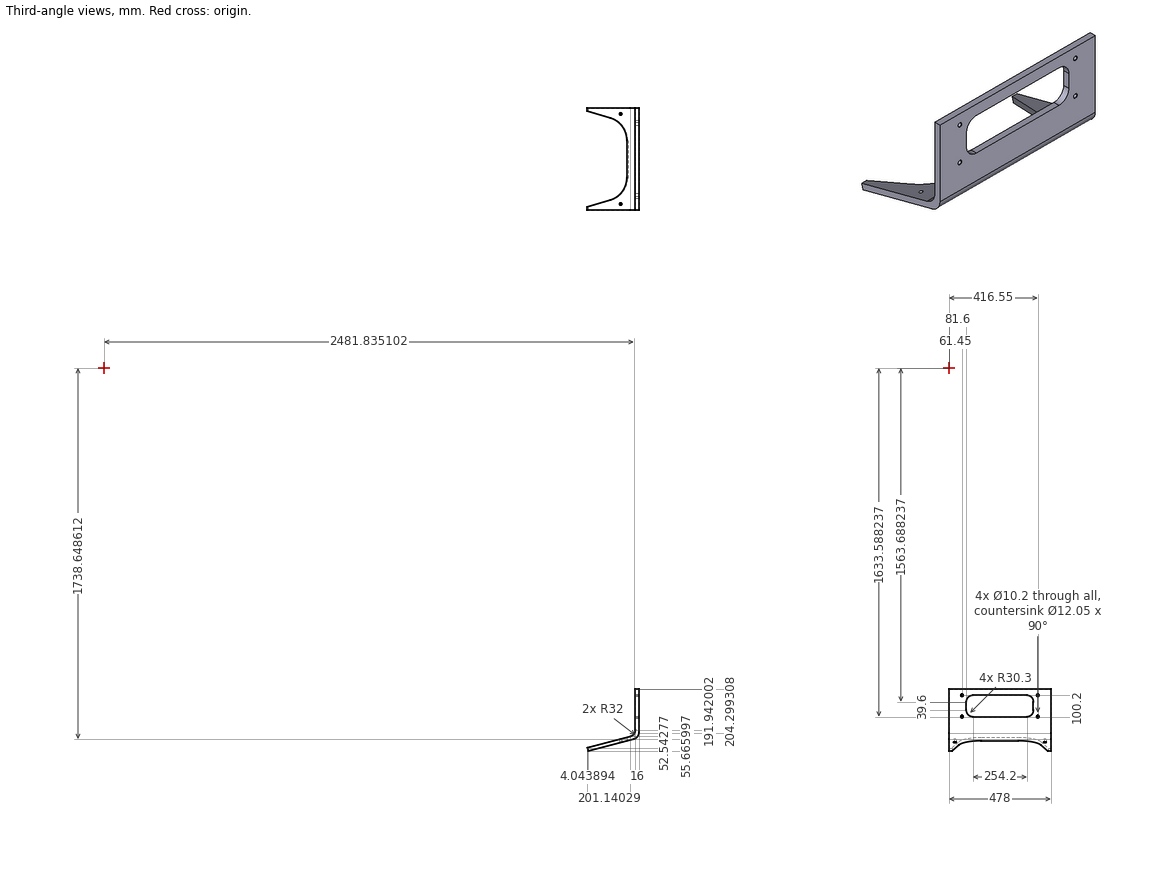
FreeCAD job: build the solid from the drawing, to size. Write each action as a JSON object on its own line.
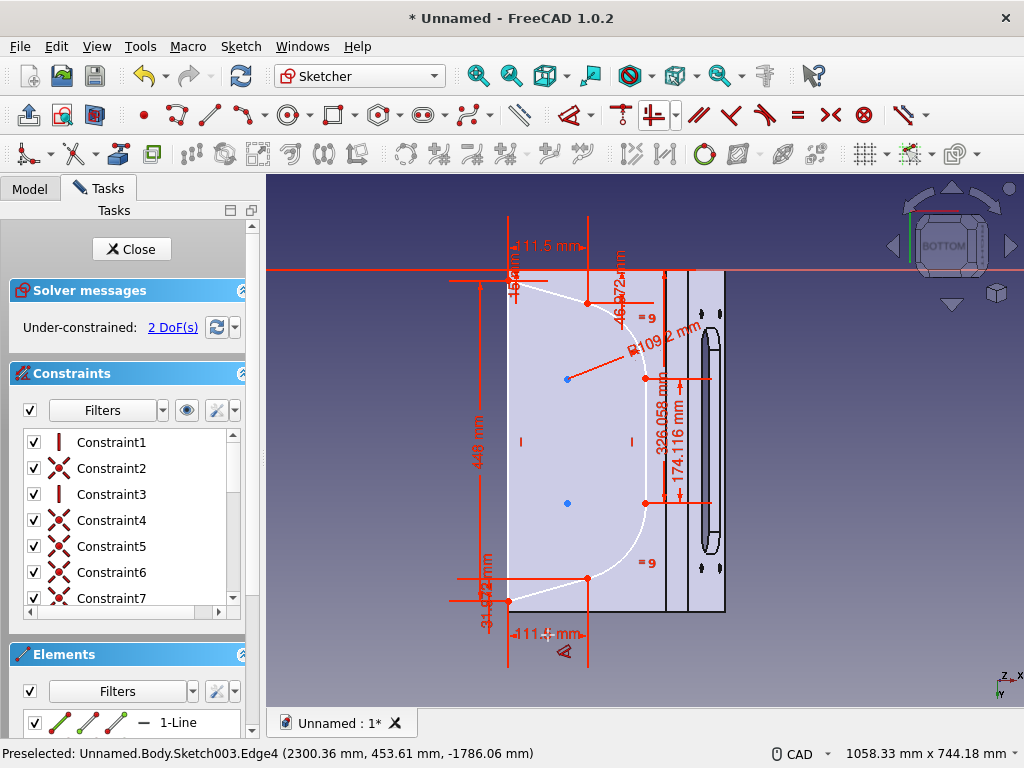
{"action": "left_click", "coordinate": [568, 379]}
{"action": "left_click", "coordinate": [602, 363]}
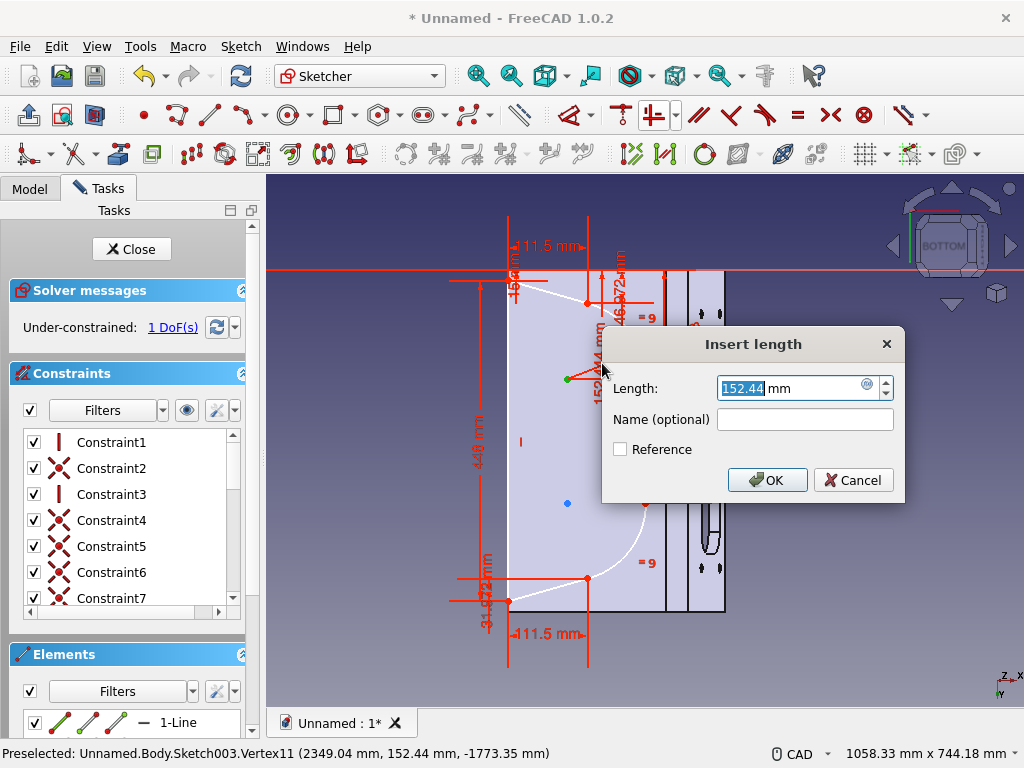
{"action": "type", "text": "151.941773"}
{"action": "key", "text": "Return"}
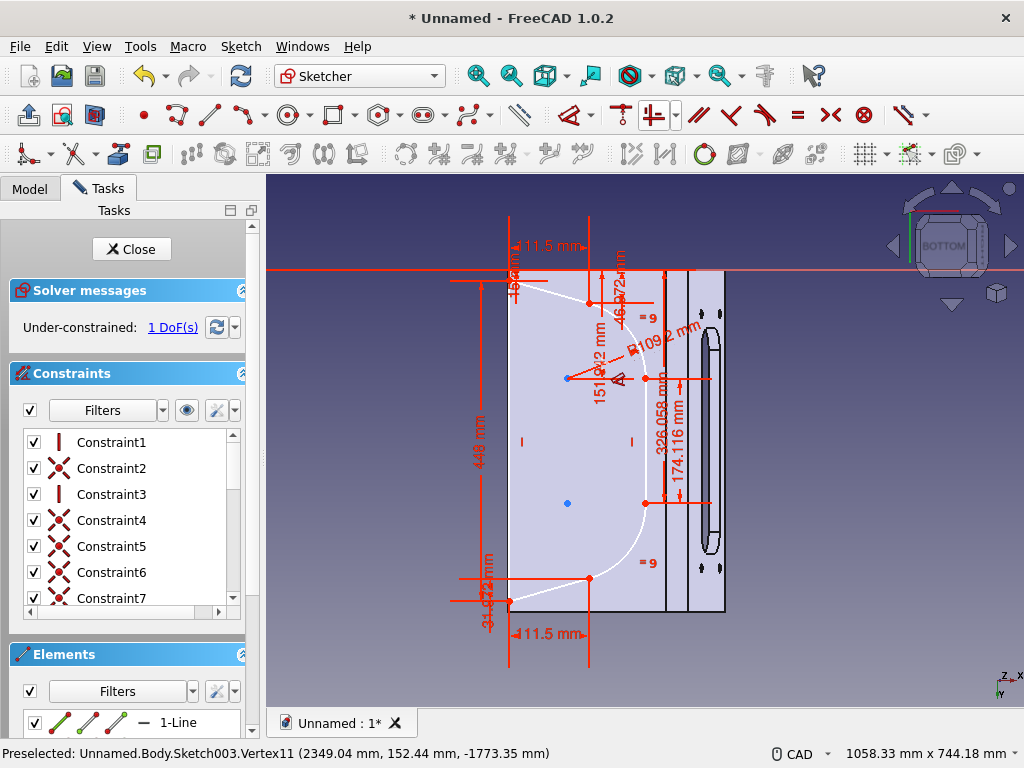
{"action": "left_click", "coordinate": [646, 503]}
{"action": "left_click", "coordinate": [470, 236]}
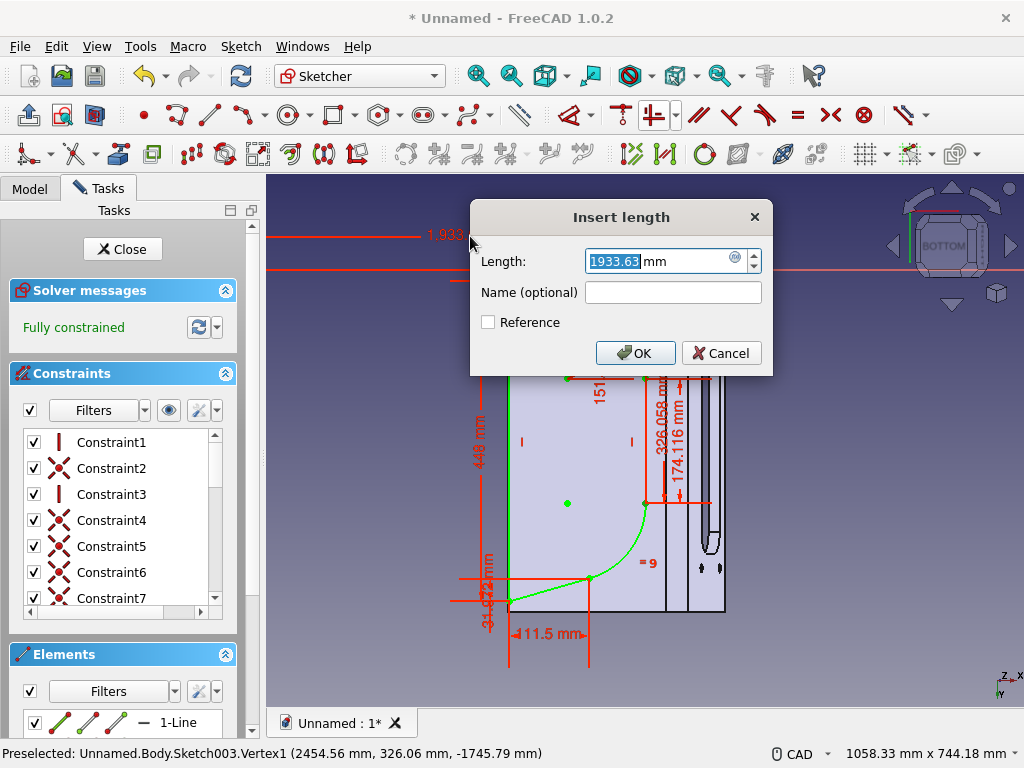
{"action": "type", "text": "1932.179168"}
{"action": "key", "text": "Return"}
{"action": "key", "text": "Escape"}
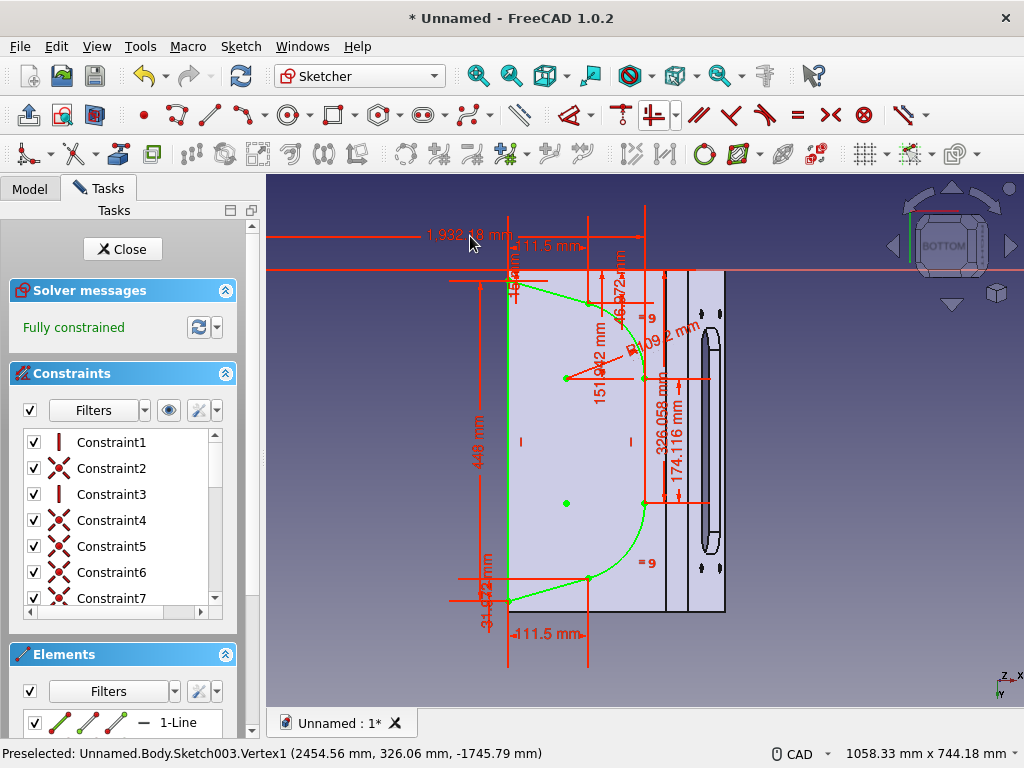
{"action": "left_click", "coordinate": [123, 249]}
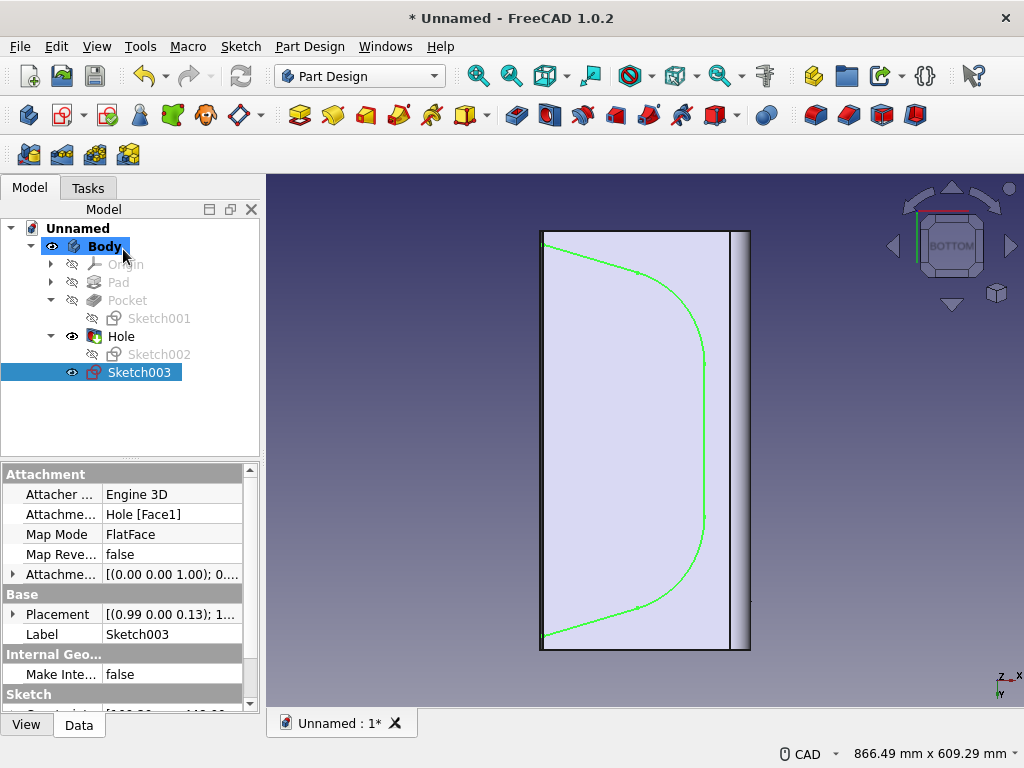
{"action": "left_click", "coordinate": [517, 116]}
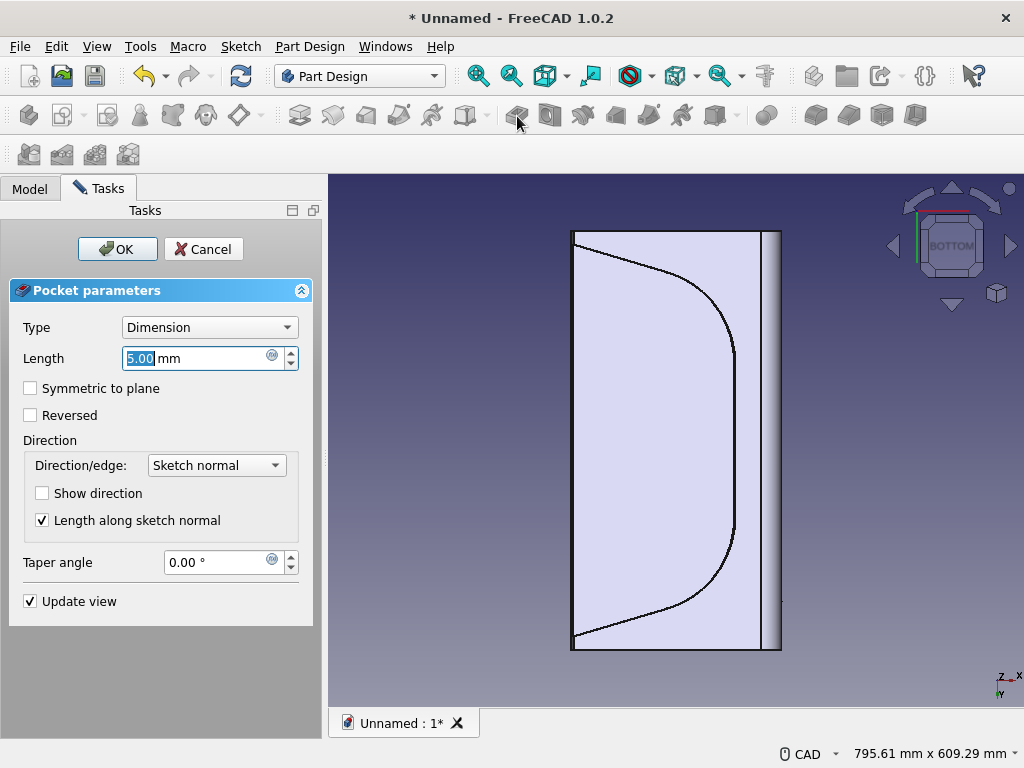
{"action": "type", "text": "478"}
{"action": "key", "text": "Tab"}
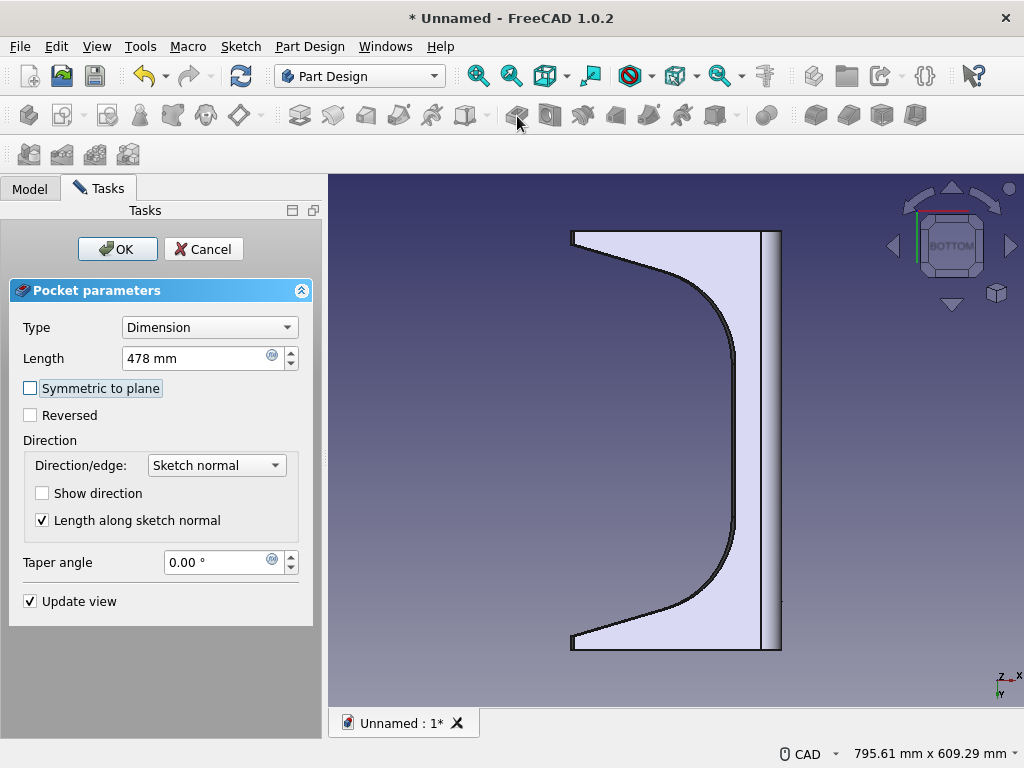
{"action": "left_click", "coordinate": [118, 249]}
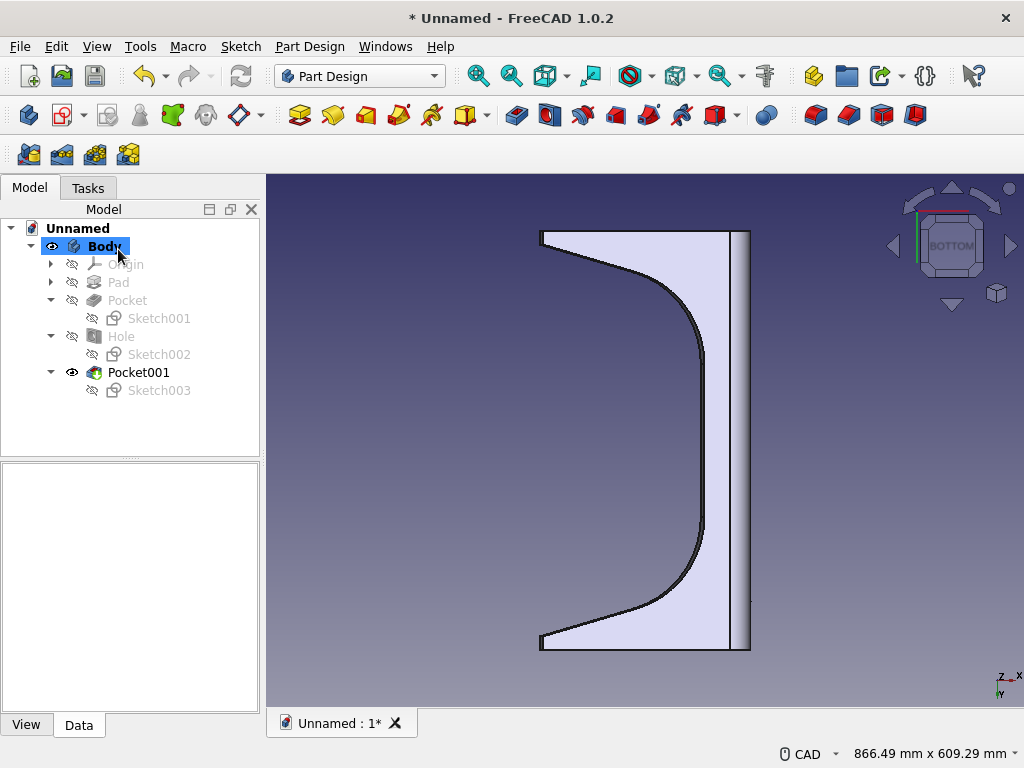
{"action": "left_click", "coordinate": [690, 260]}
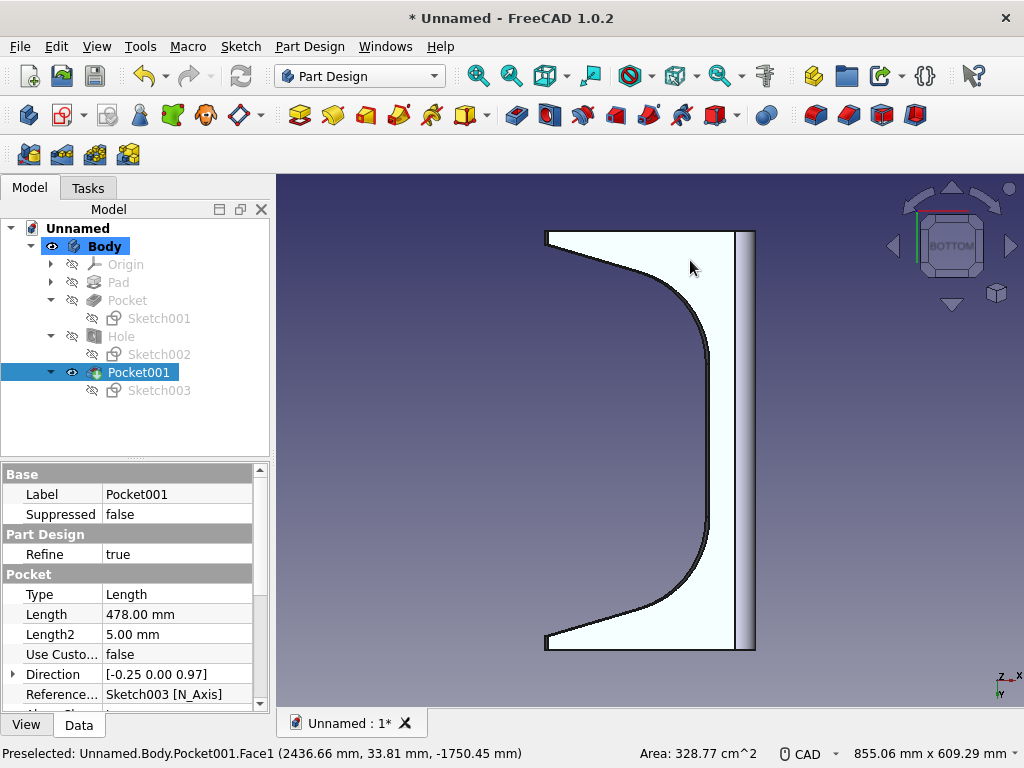
{"action": "left_click", "coordinate": [62, 116]}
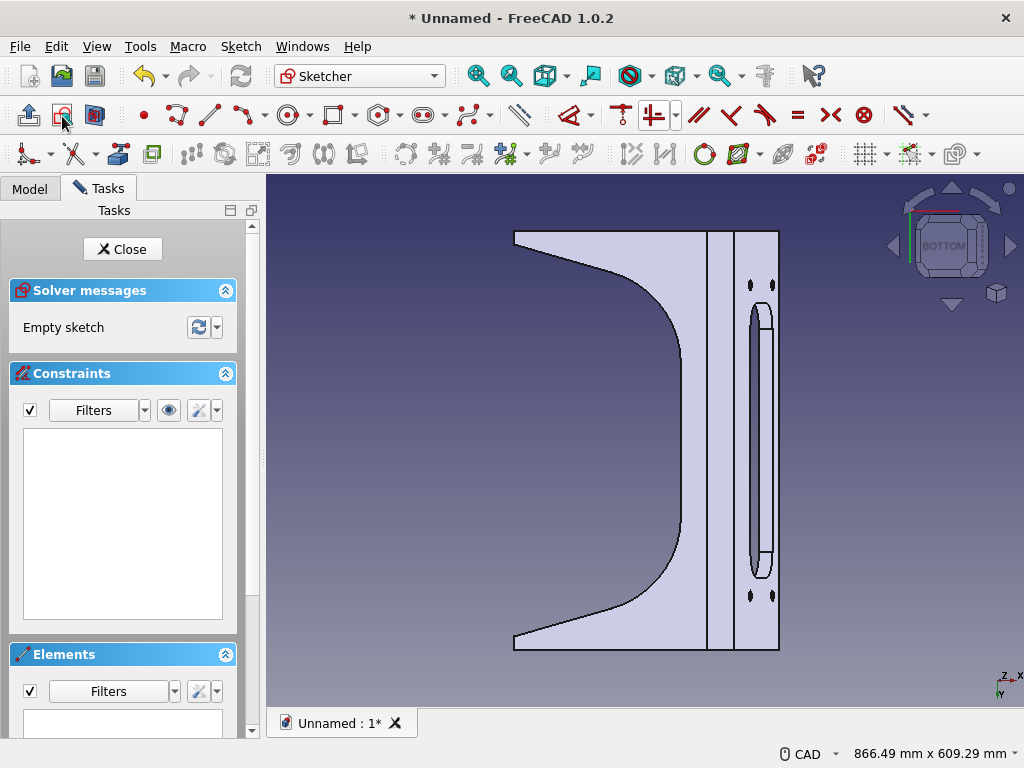
{"action": "left_click", "coordinate": [288, 116]}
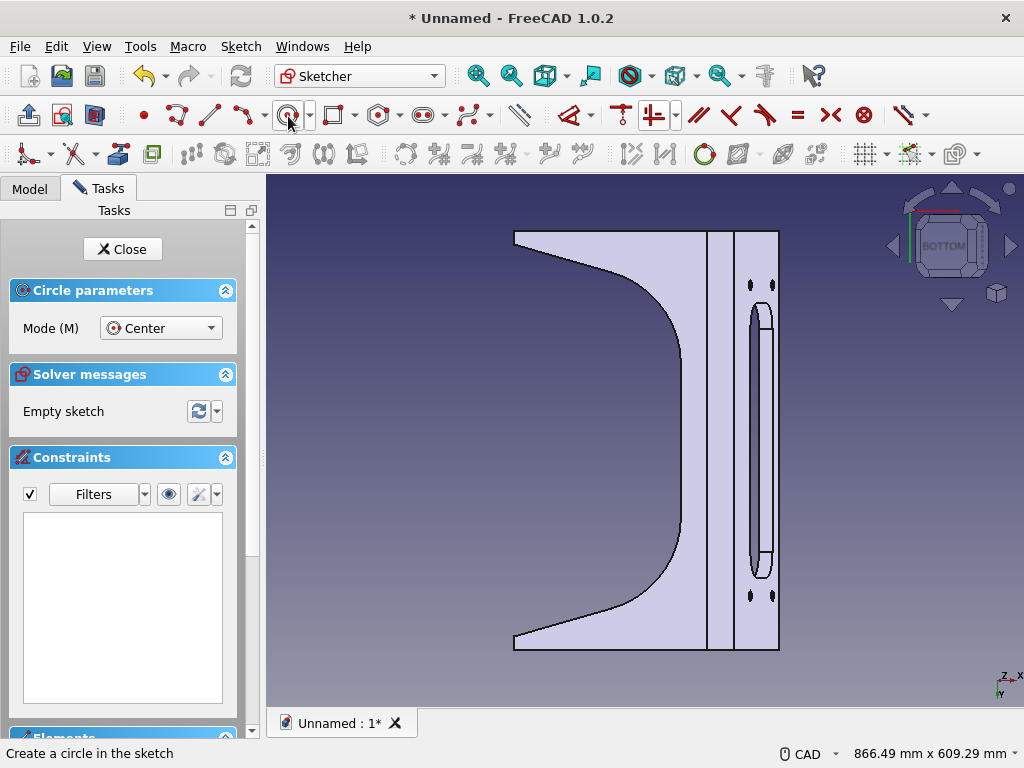
{"action": "scroll", "coordinate": [654, 625], "scroll_direction": "up", "scroll_amount": 9}